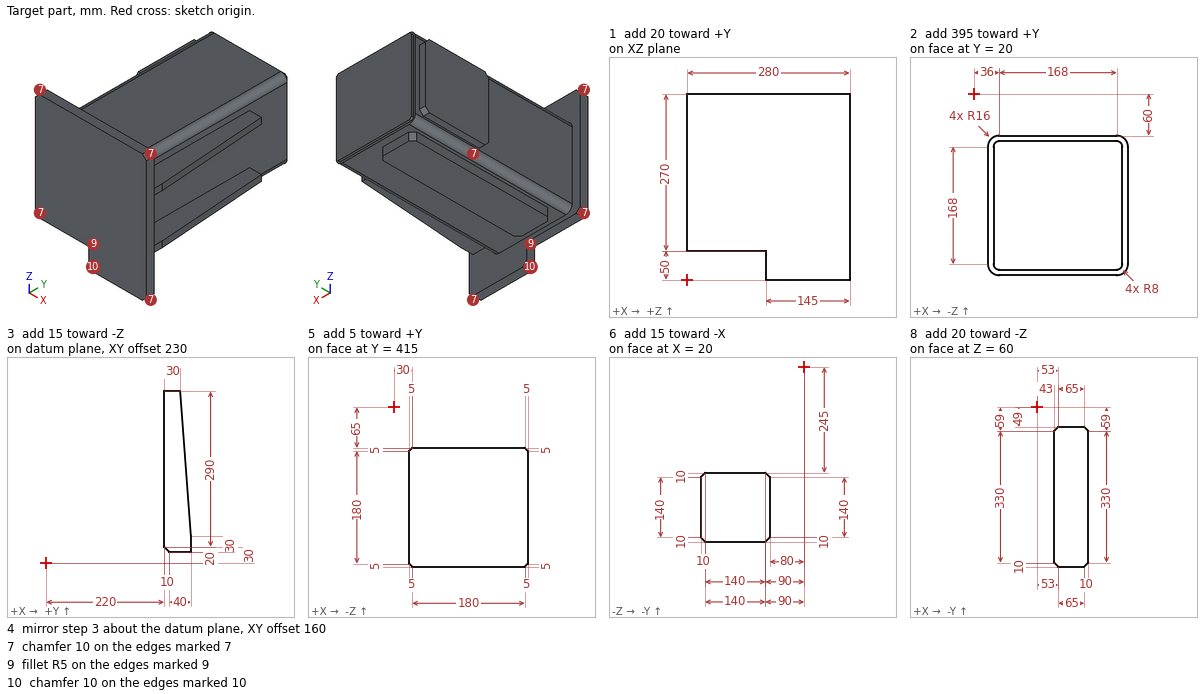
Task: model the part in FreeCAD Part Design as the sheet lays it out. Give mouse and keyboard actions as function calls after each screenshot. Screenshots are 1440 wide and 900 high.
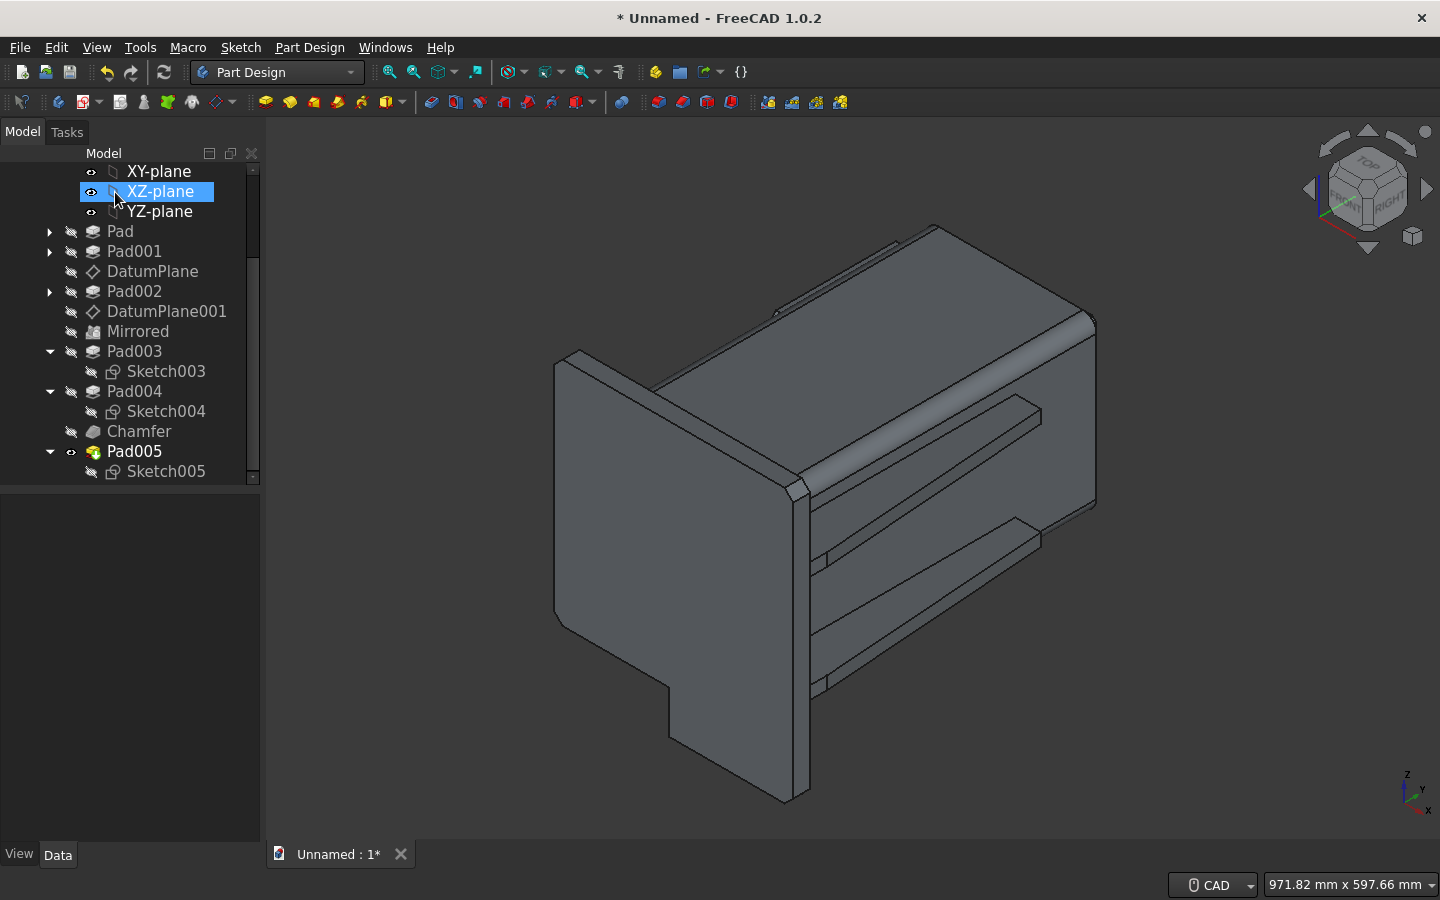
key(2)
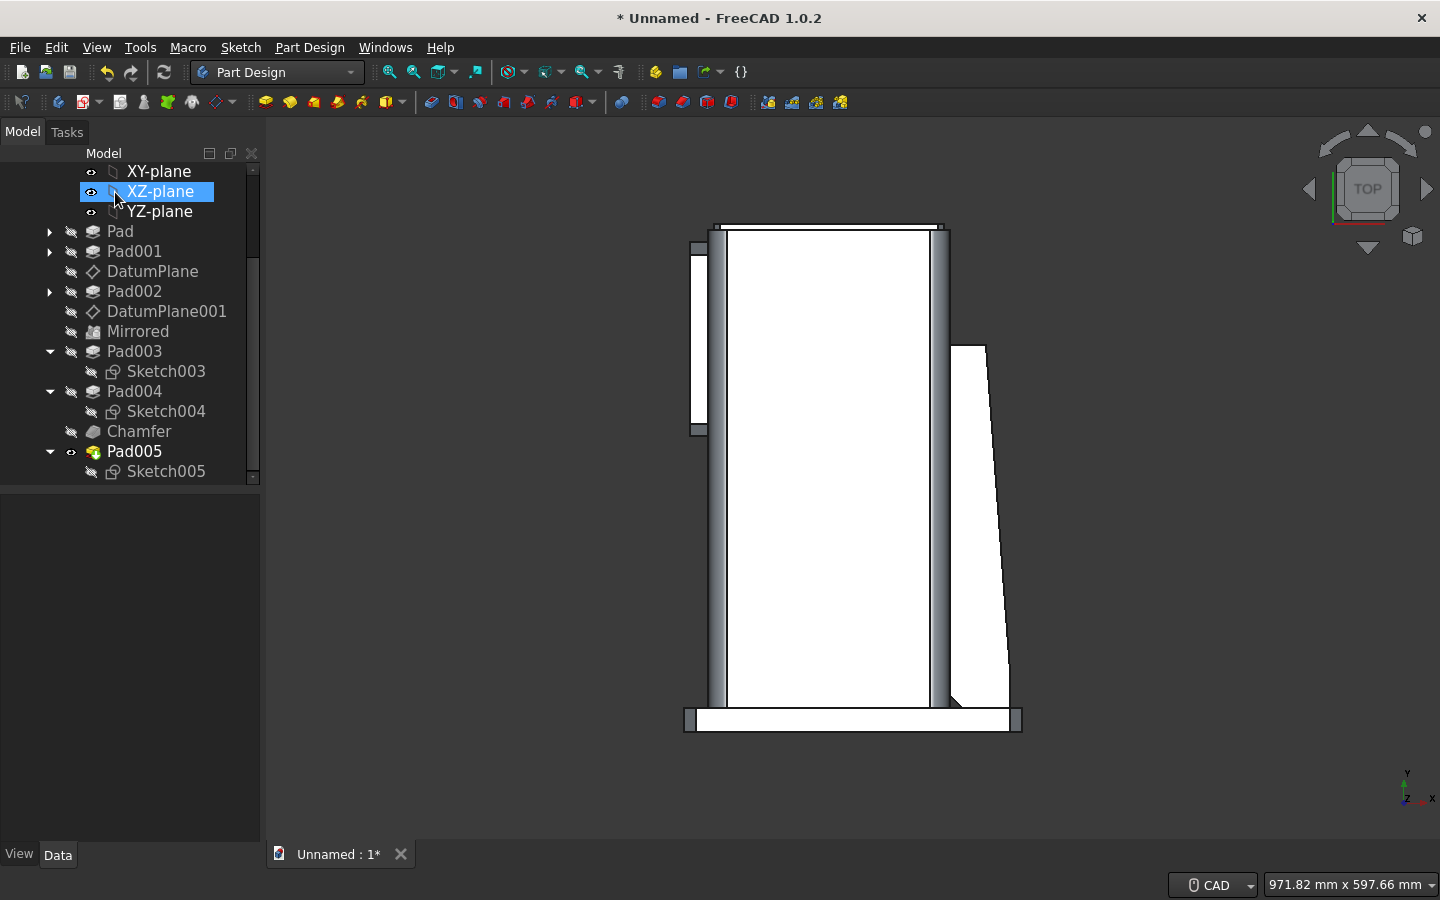
key(1)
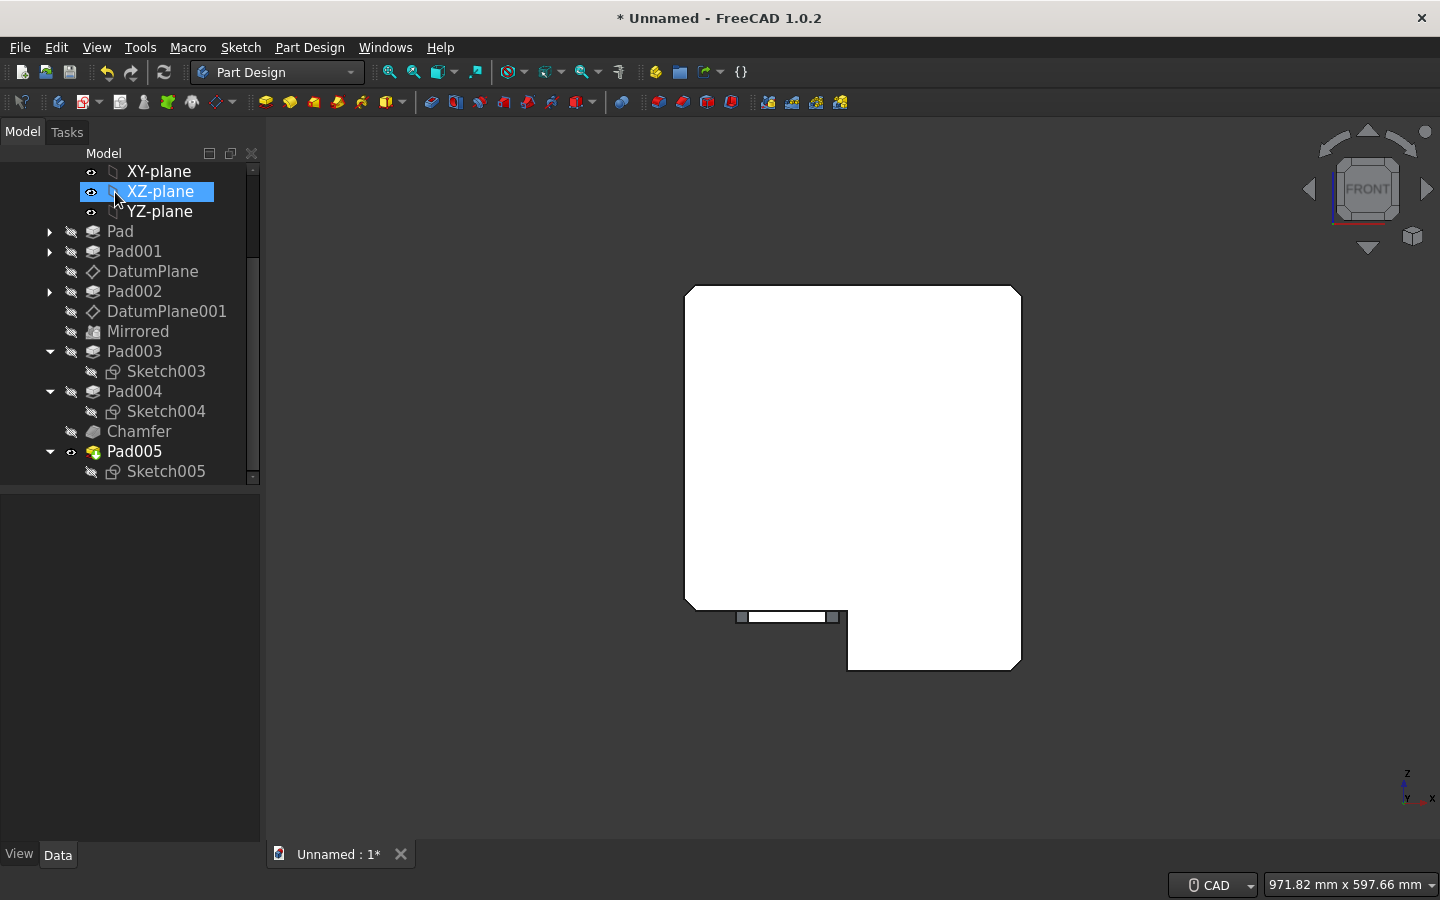
key(3)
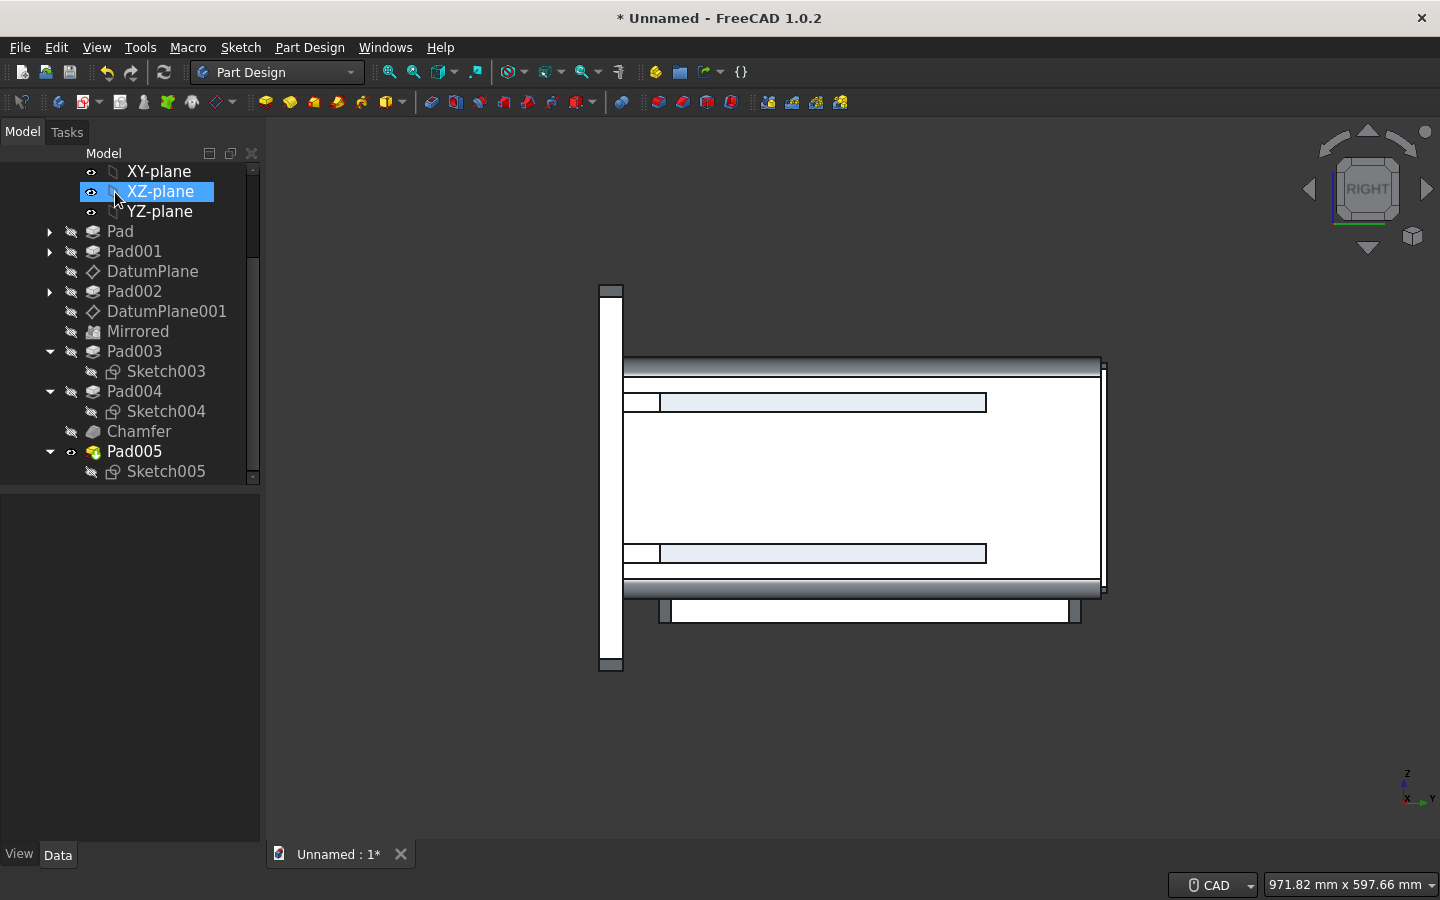
key(5)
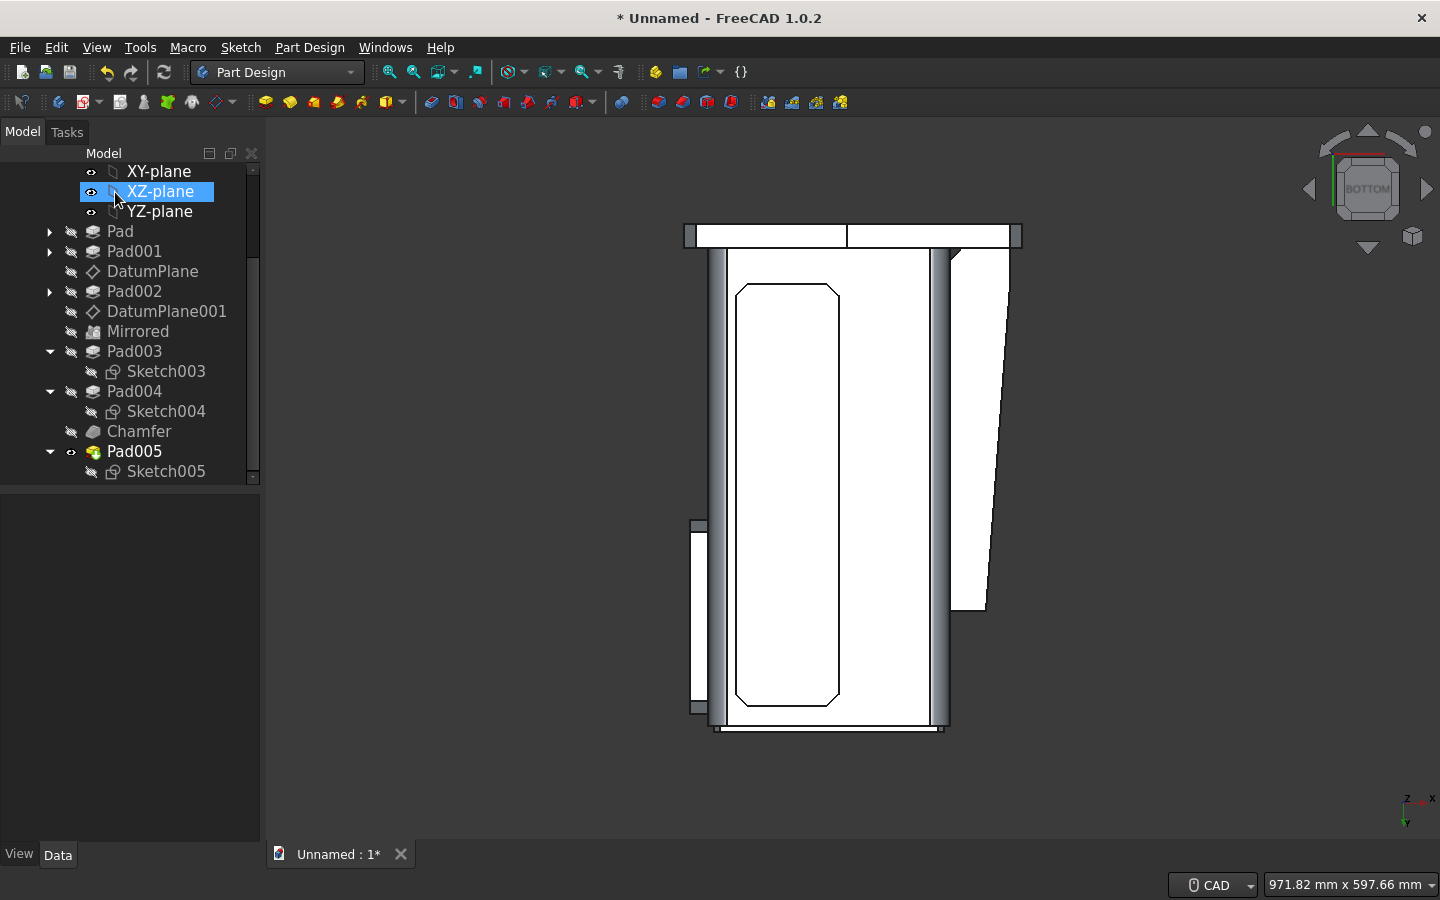
key(4)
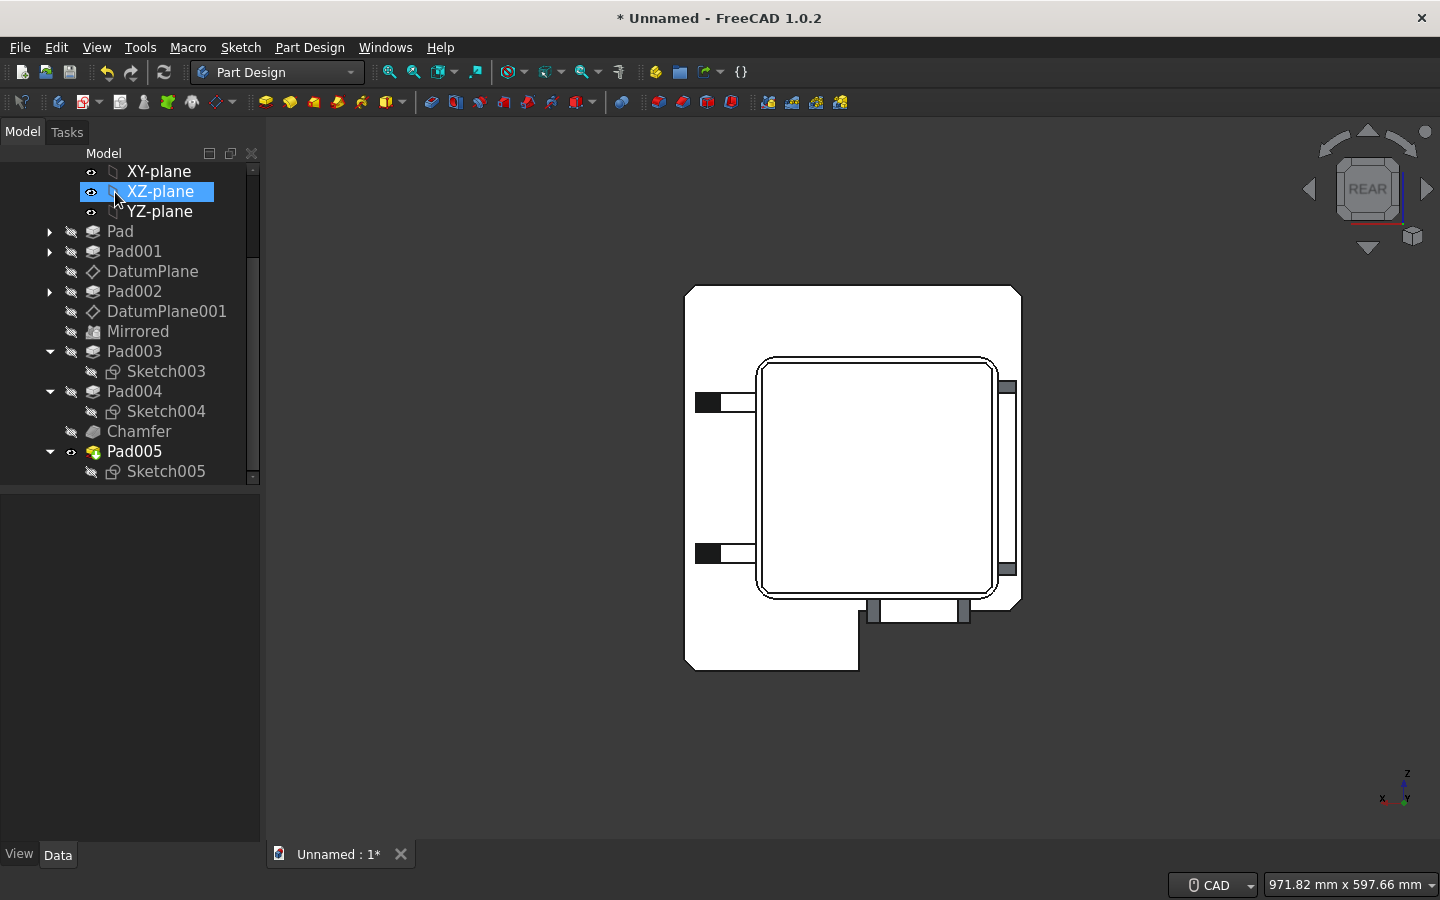
key(6)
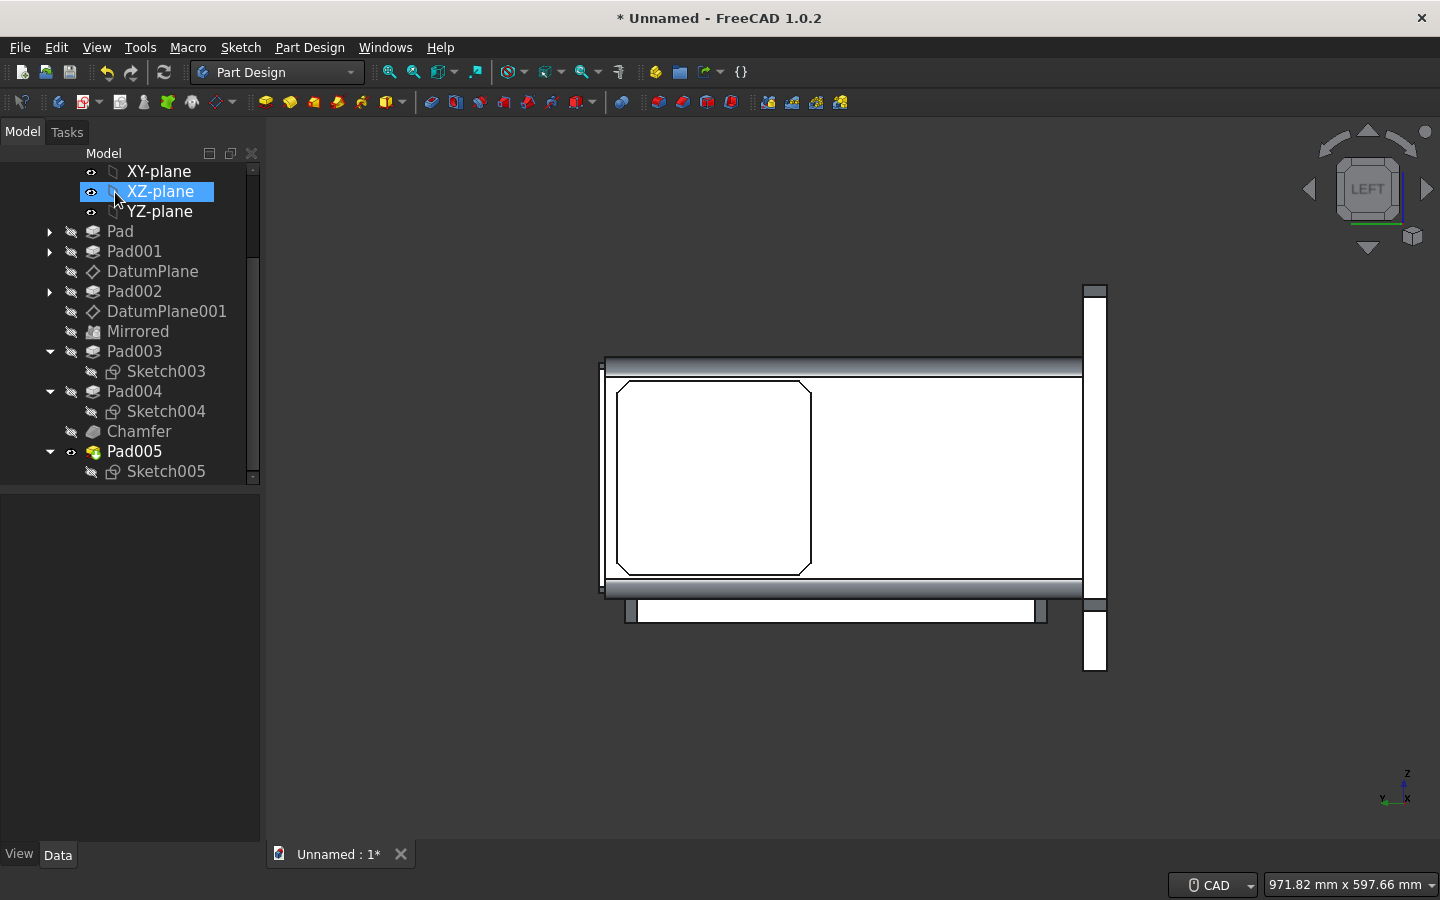
key(v)
key(3)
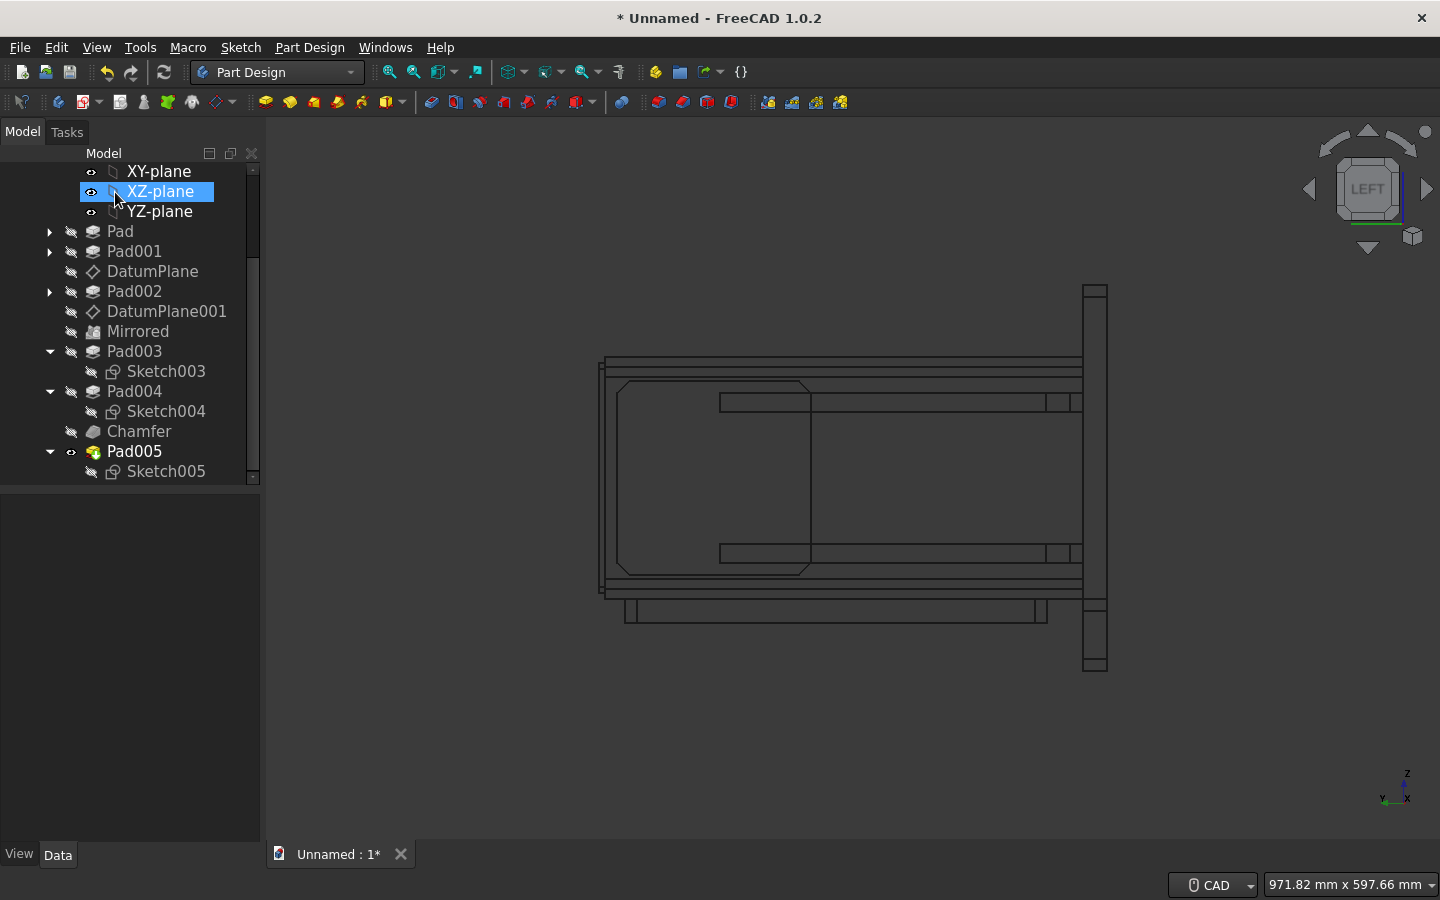
key(0)